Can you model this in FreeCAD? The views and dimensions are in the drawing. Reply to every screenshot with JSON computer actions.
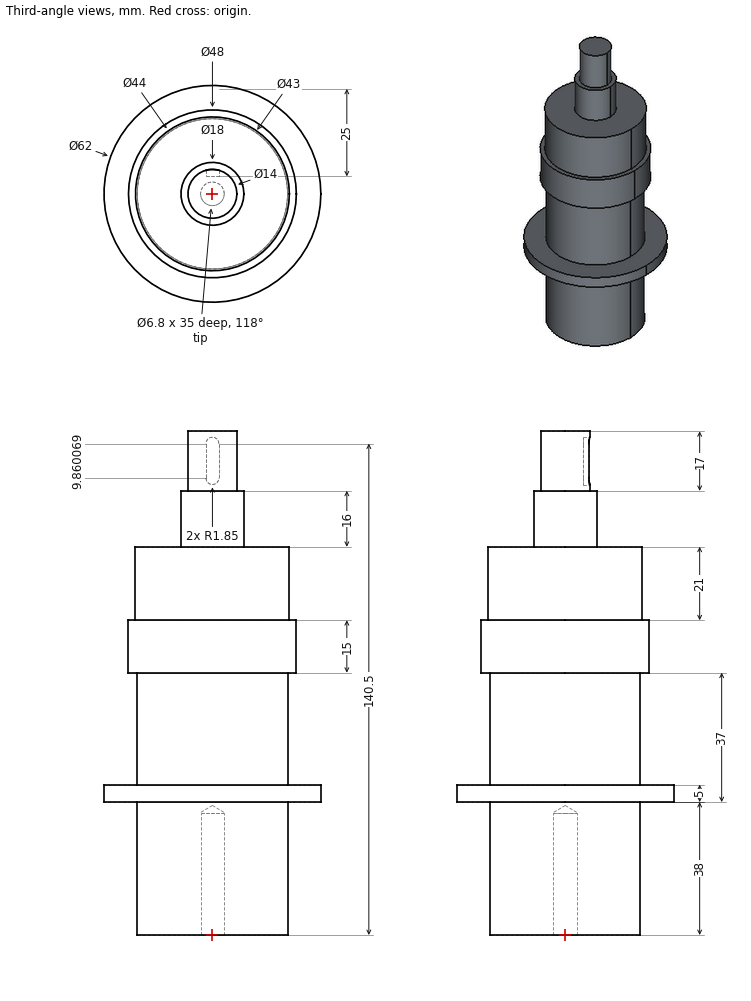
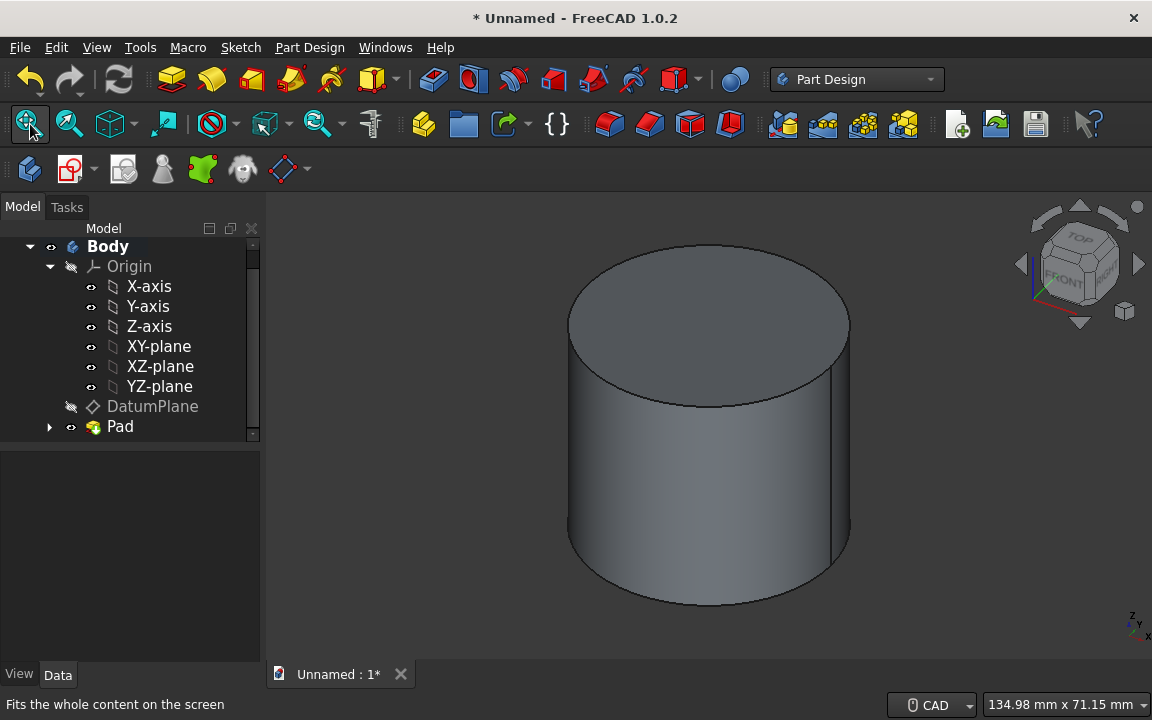
{"action": "left_click", "coordinate": [709, 325]}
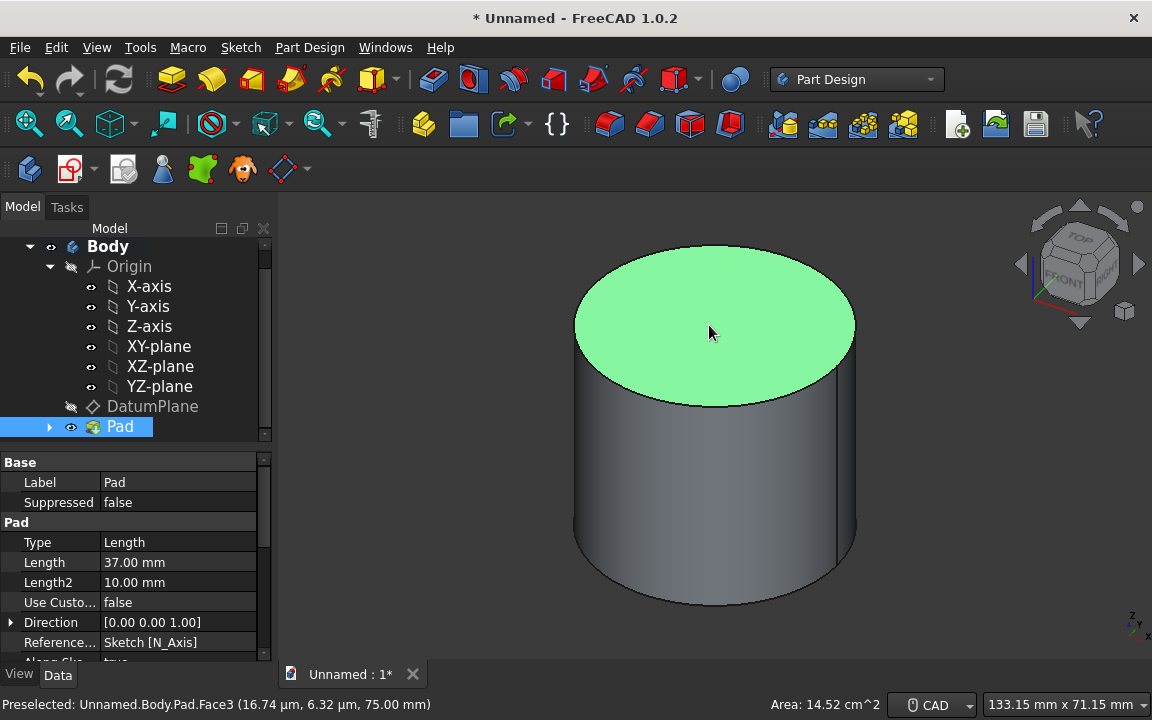
{"action": "left_click", "coordinate": [70, 170]}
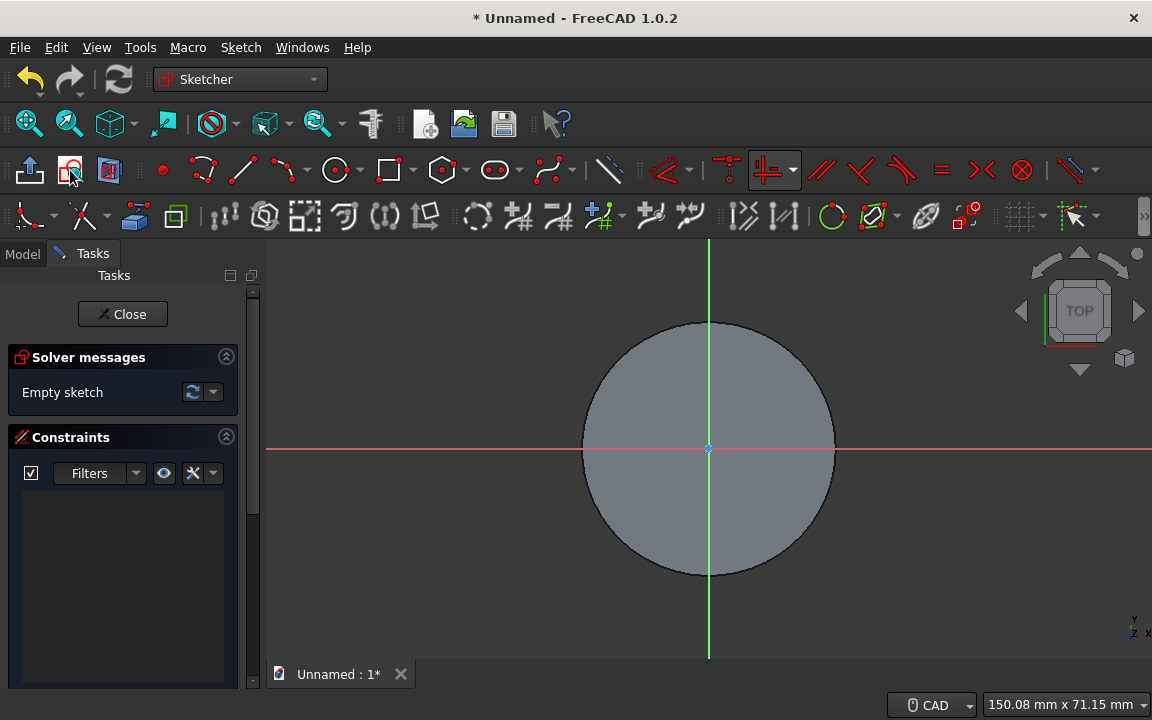
{"action": "key", "text": "g c"}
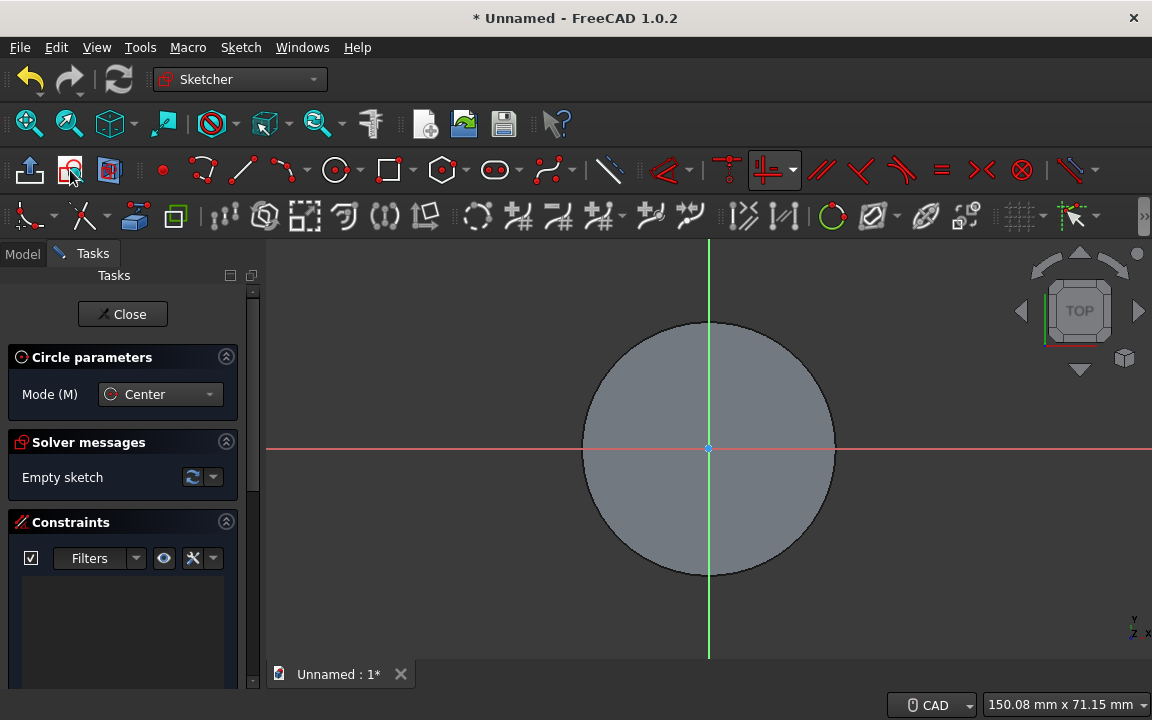
{"action": "left_click", "coordinate": [709, 449]}
{"action": "left_click", "coordinate": [809, 349]}
{"action": "key", "text": "Escape"}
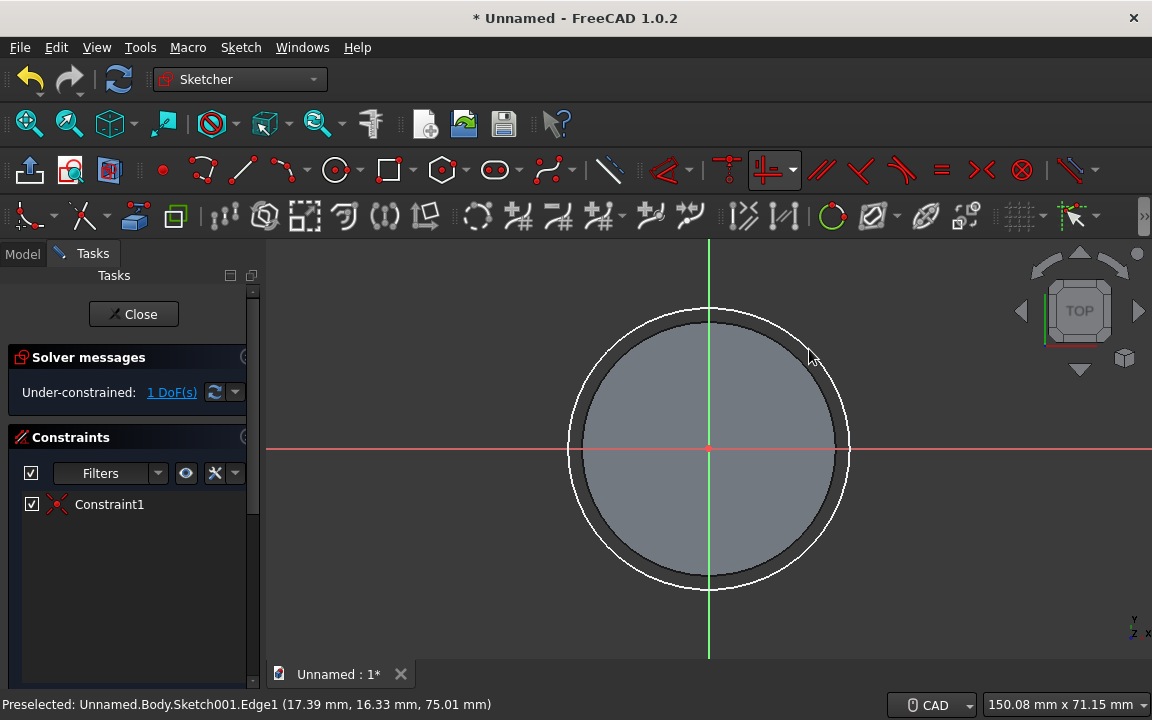
{"action": "left_click", "coordinate": [664, 170]}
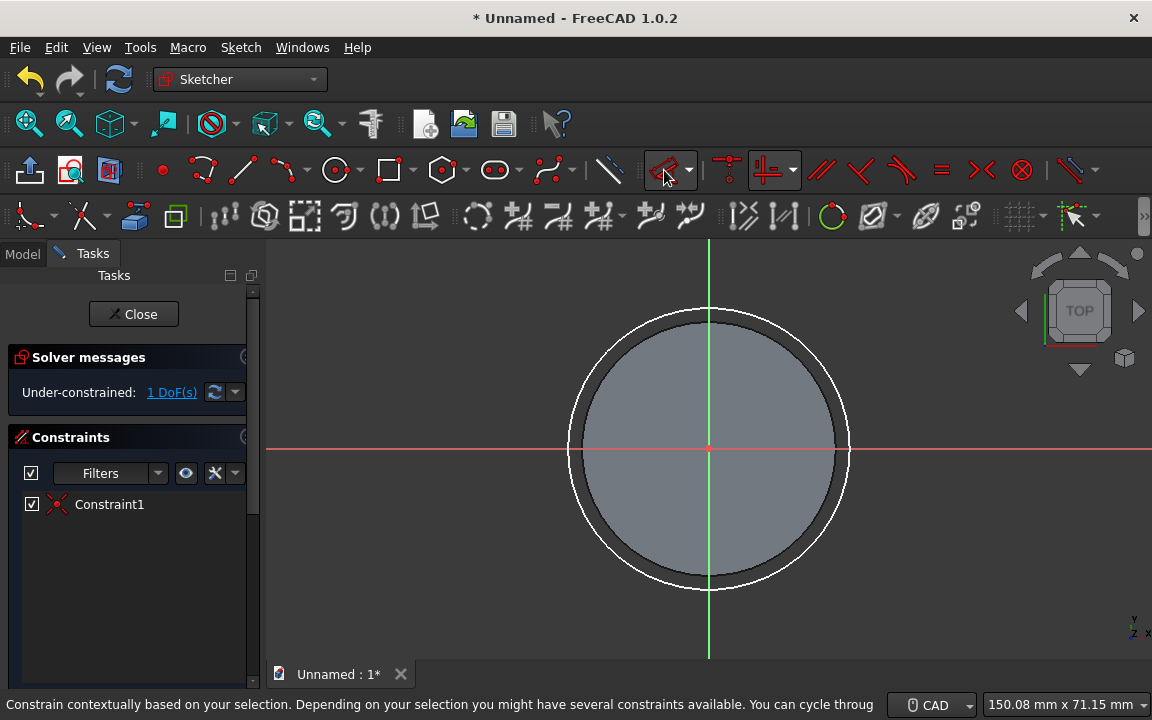
{"action": "left_click", "coordinate": [808, 349]}
{"action": "left_click", "coordinate": [831, 326]}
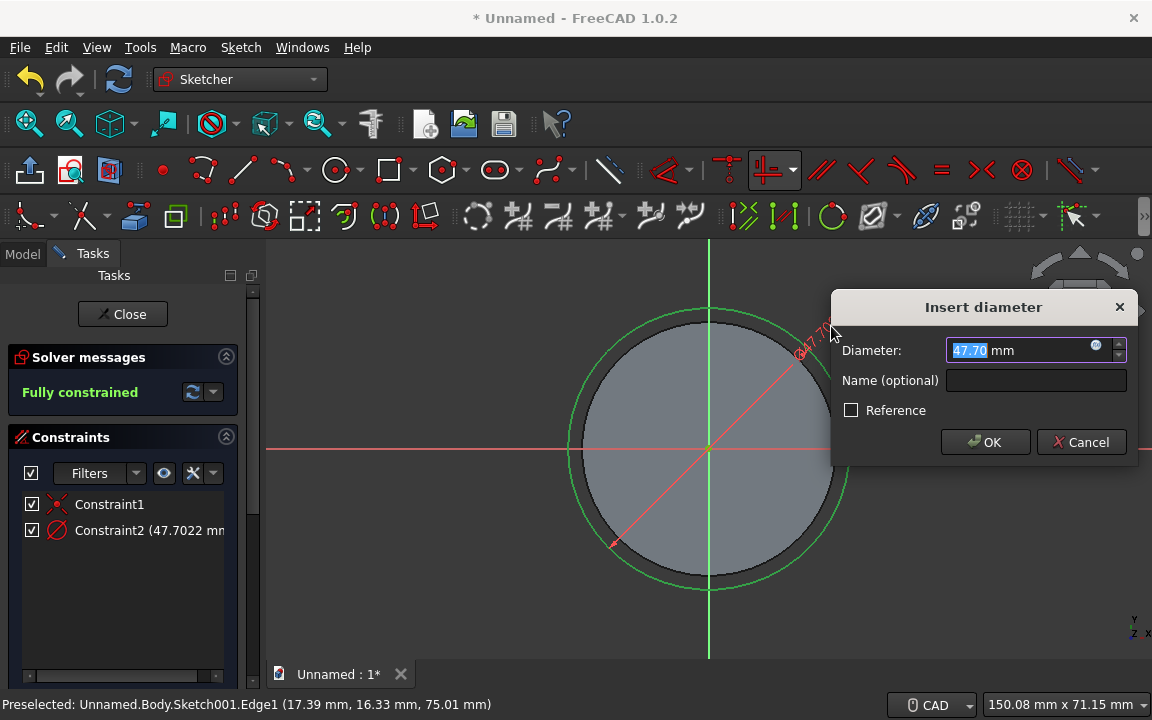
{"action": "type", "text": "48"}
{"action": "key", "text": "Return"}
{"action": "key", "text": "Escape"}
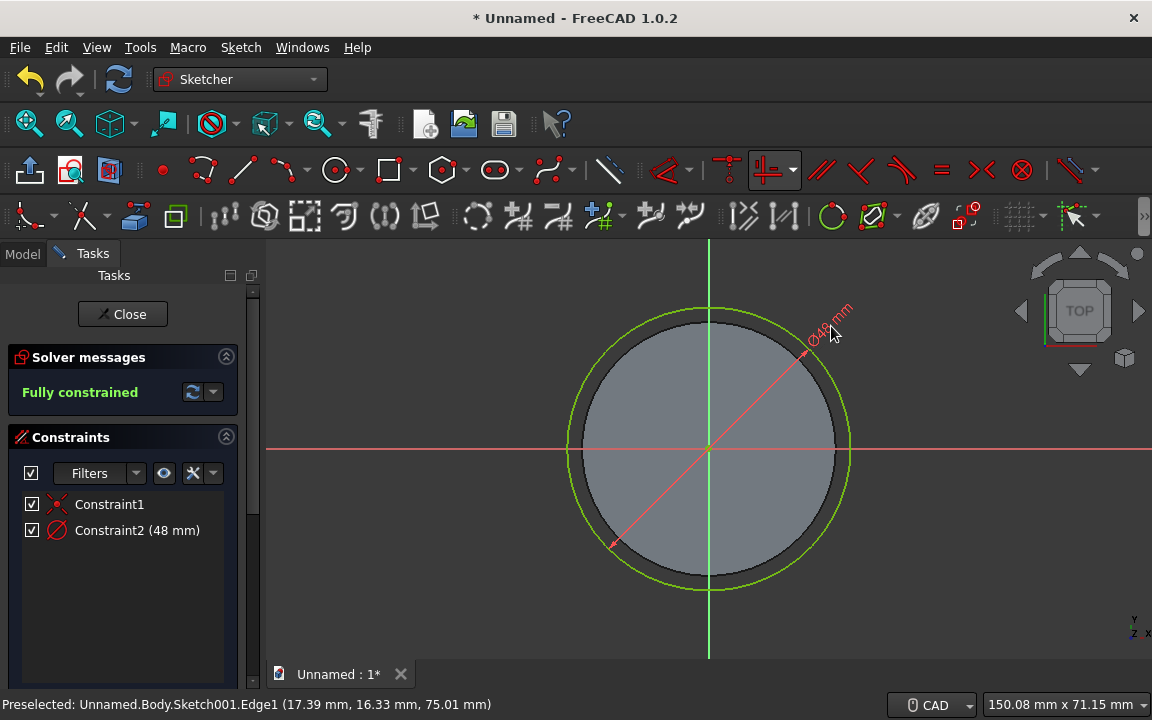
{"action": "left_click", "coordinate": [123, 314]}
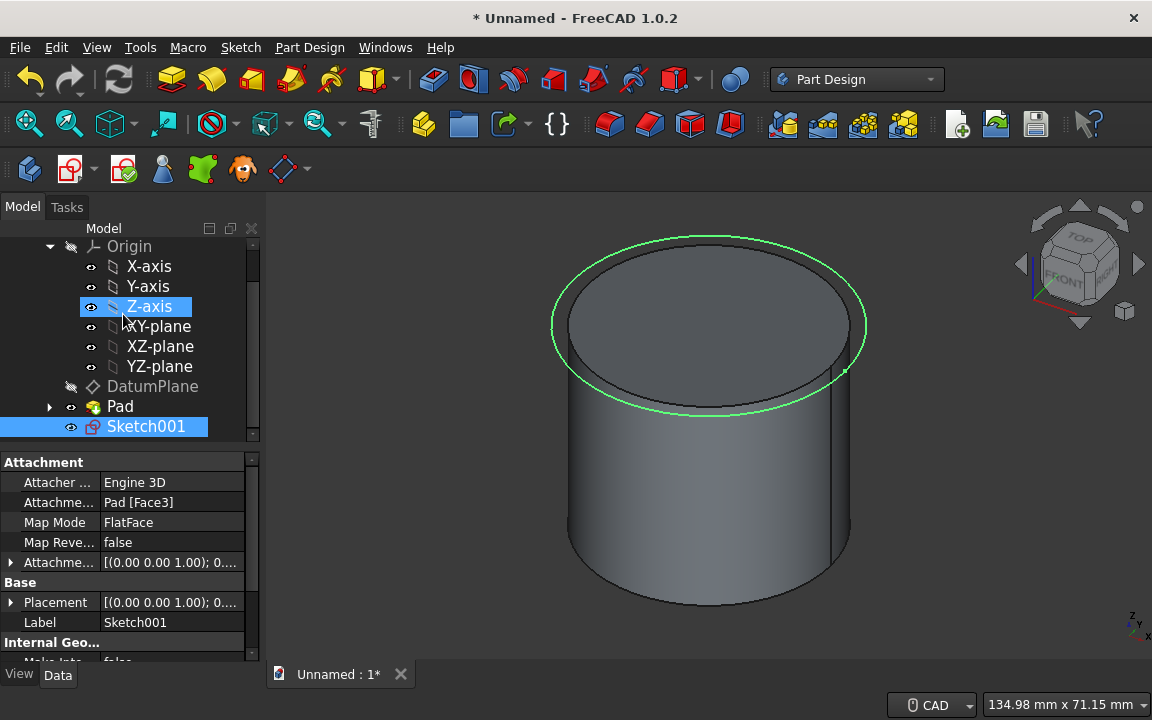
{"action": "left_click", "coordinate": [172, 80]}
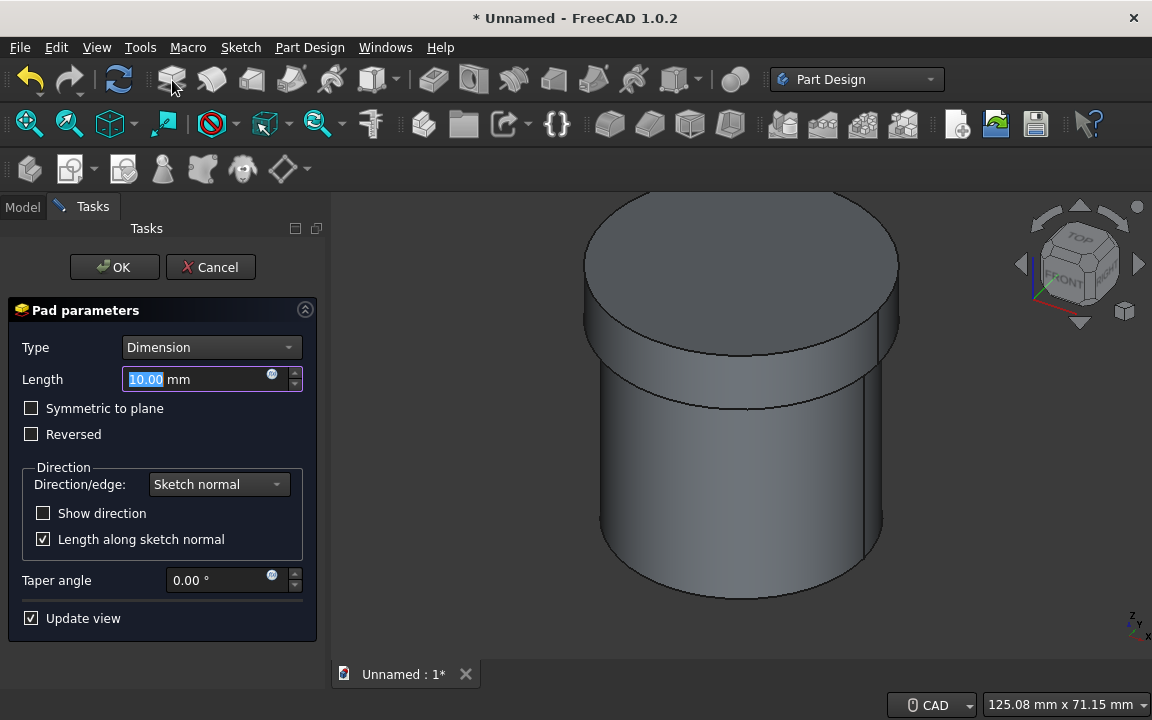
{"action": "type", "text": "15"}
{"action": "key", "text": "Tab"}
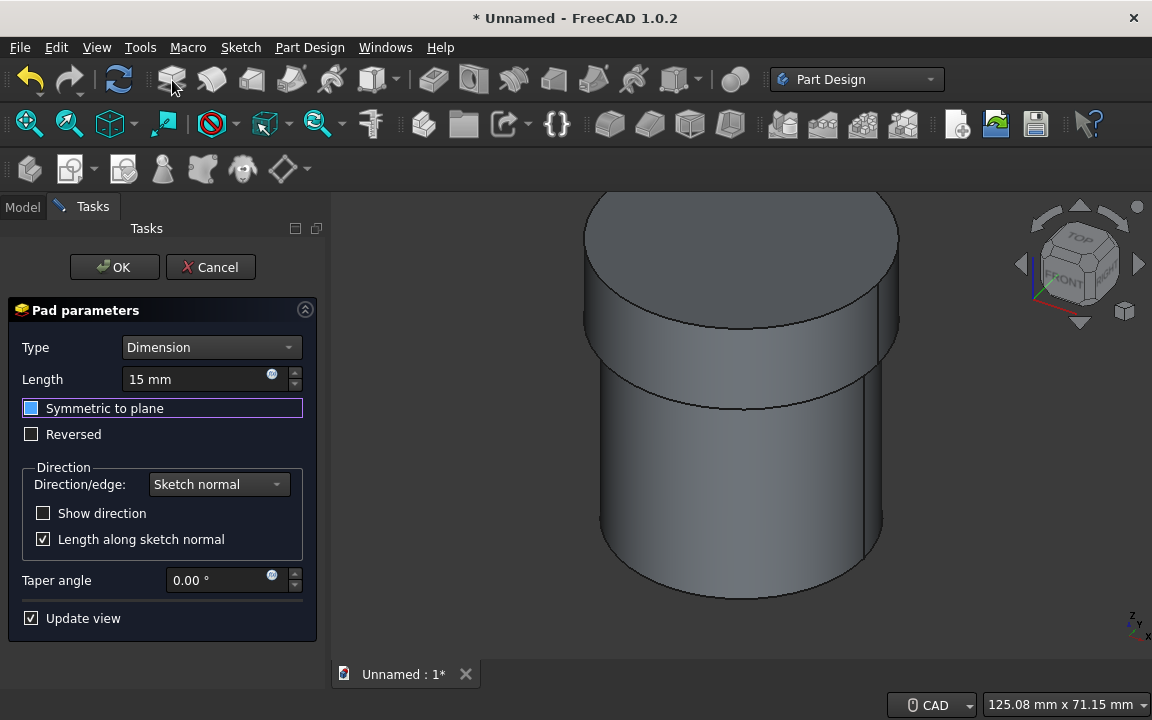
{"action": "left_click", "coordinate": [115, 267]}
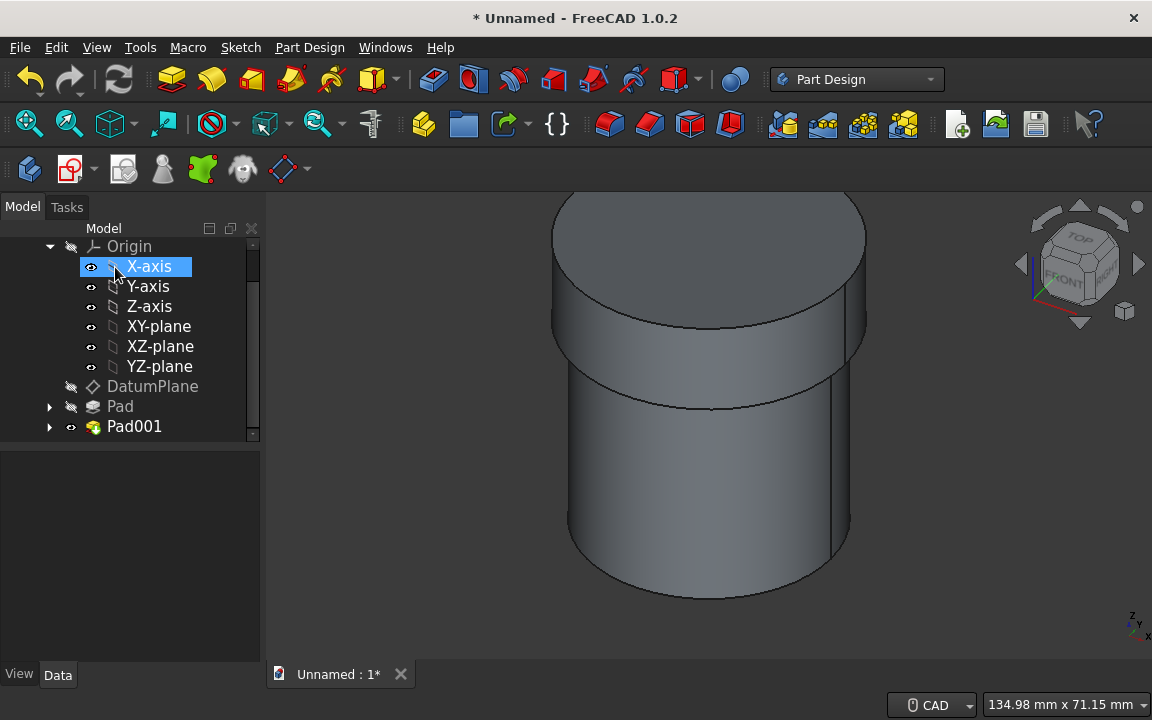
{"action": "left_click", "coordinate": [30, 124]}